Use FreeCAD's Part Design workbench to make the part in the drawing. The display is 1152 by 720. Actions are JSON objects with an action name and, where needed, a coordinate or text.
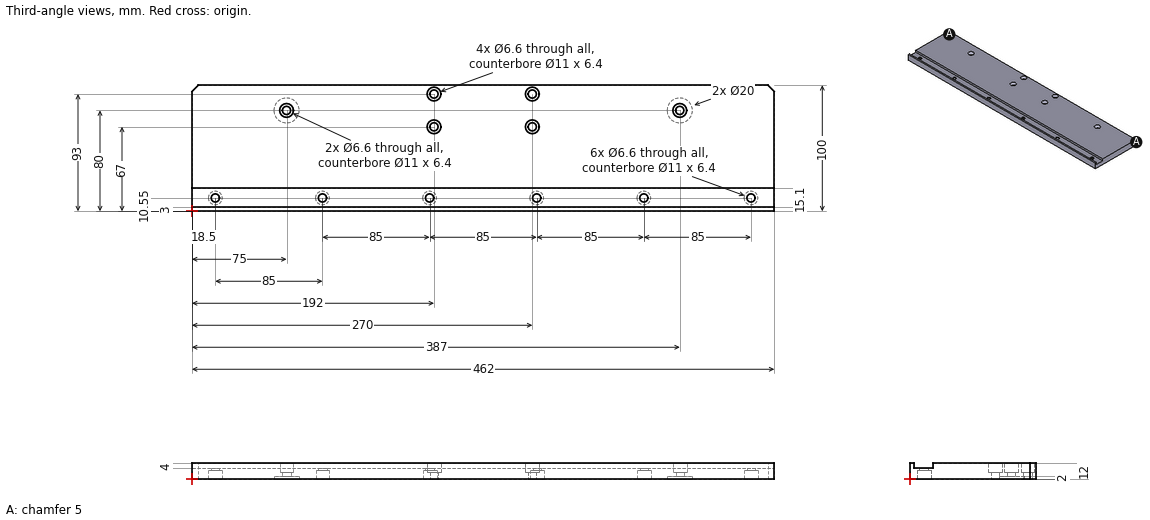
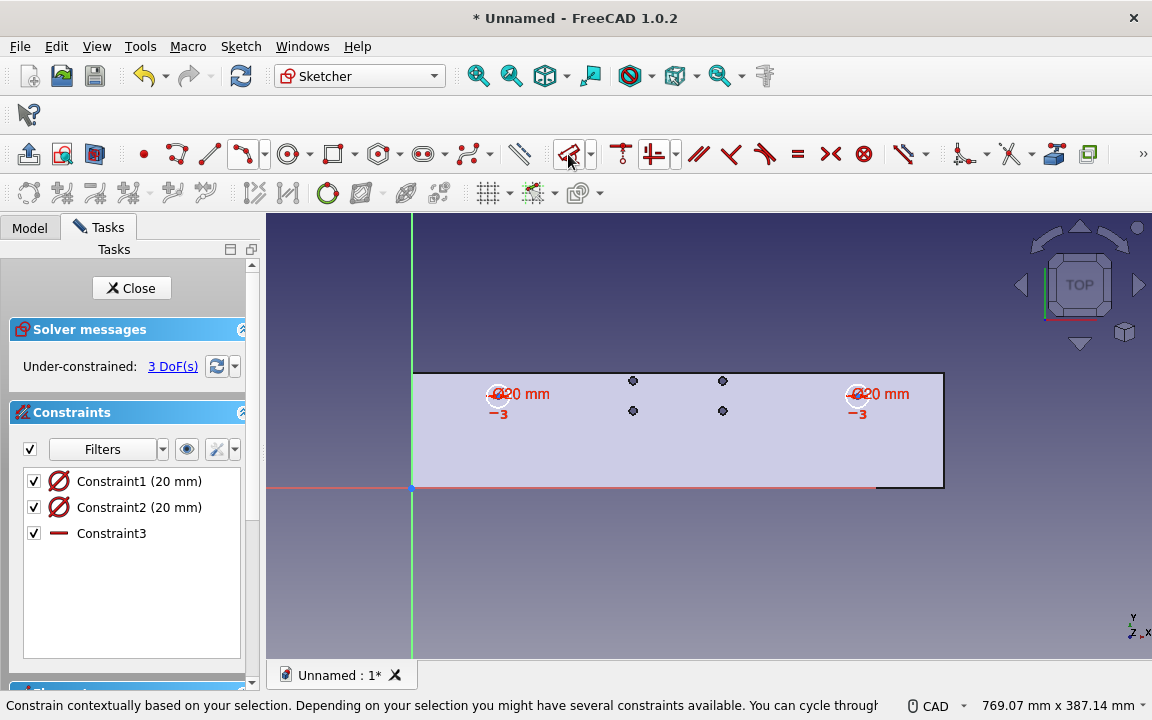
{"action": "left_click", "coordinate": [858, 396]}
{"action": "left_click", "coordinate": [378, 442]}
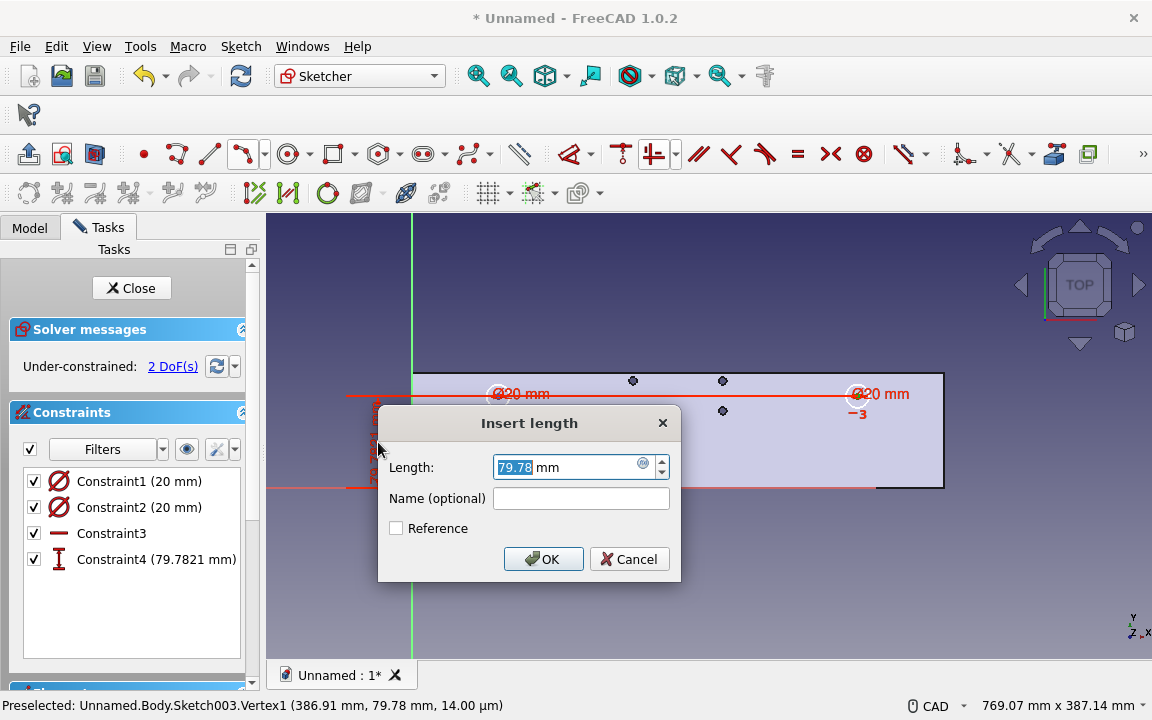
{"action": "type", "text": "80"}
{"action": "key", "text": "Return"}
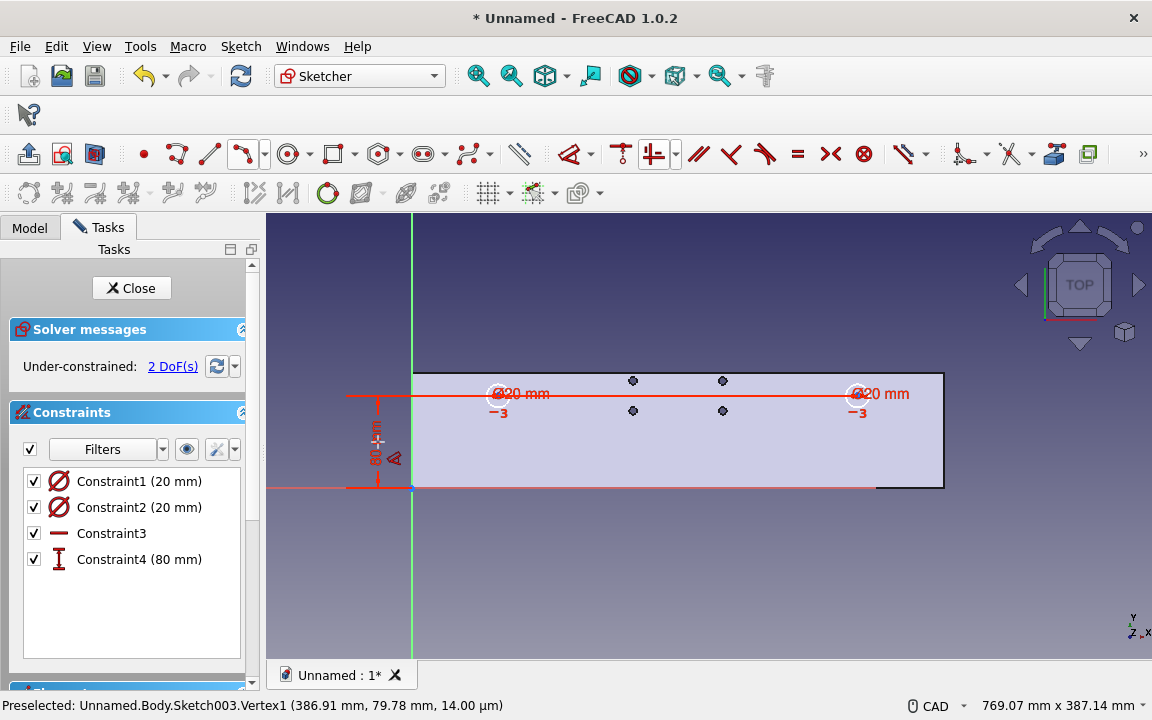
{"action": "left_click", "coordinate": [498, 396]}
{"action": "left_click", "coordinate": [455, 522]}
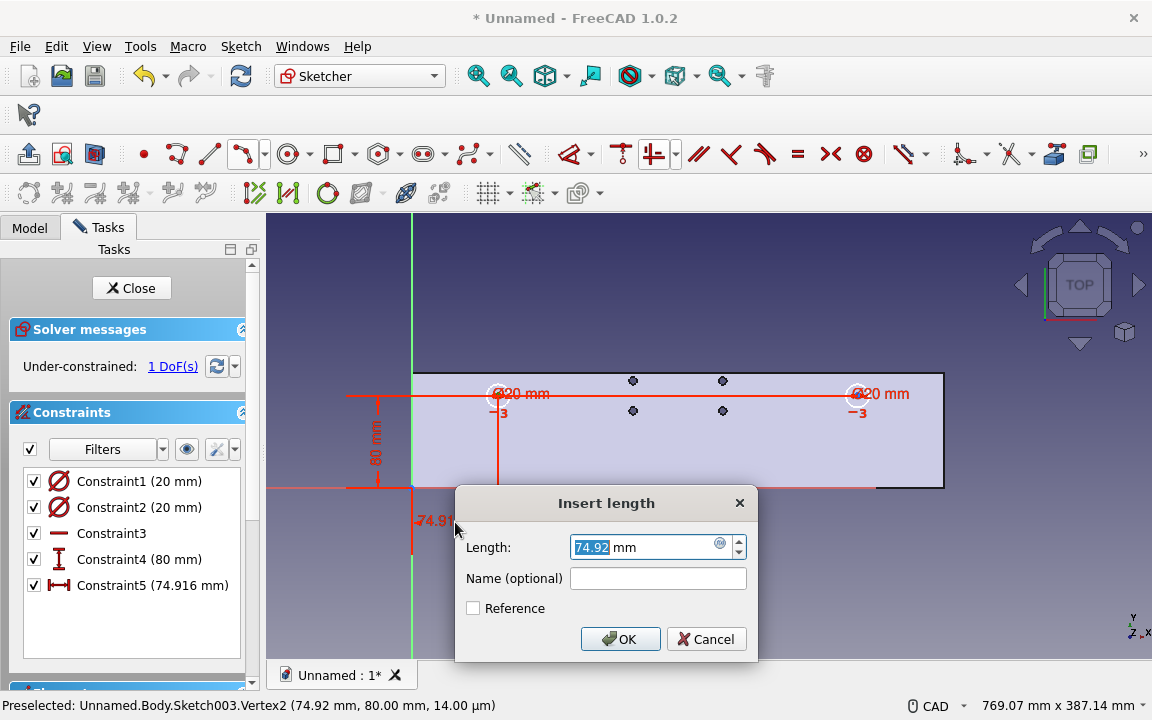
{"action": "type", "text": "75"}
{"action": "key", "text": "Return"}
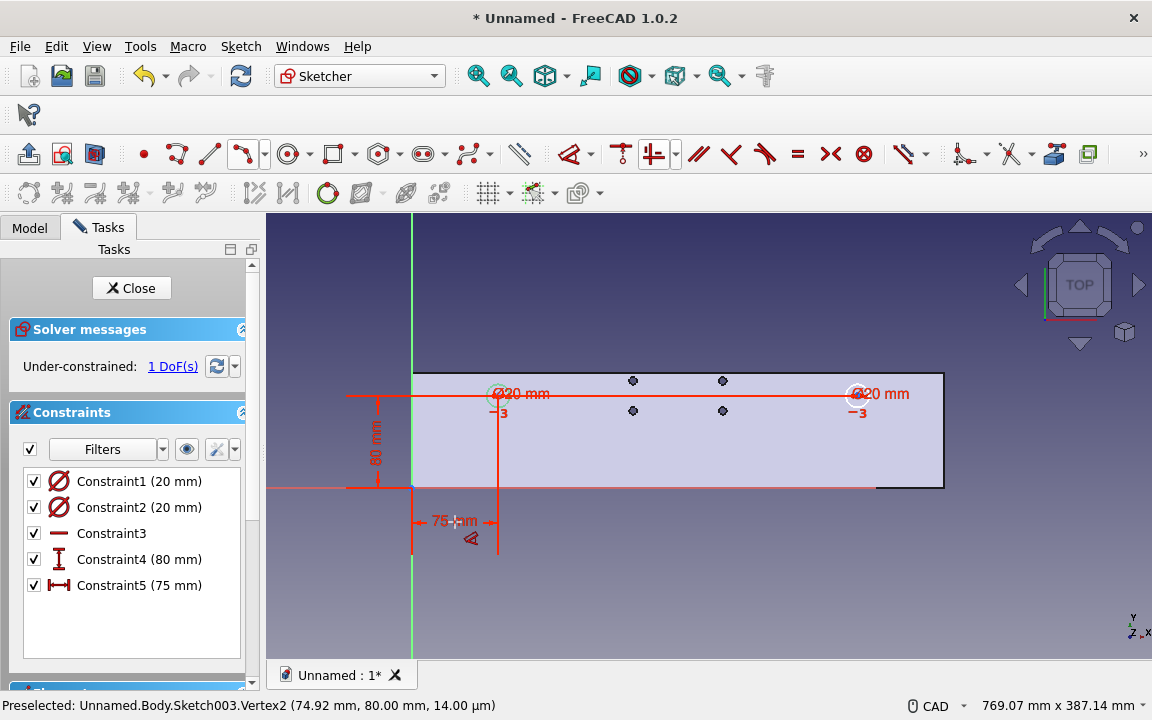
{"action": "left_click", "coordinate": [858, 396]}
{"action": "left_click", "coordinate": [635, 522]}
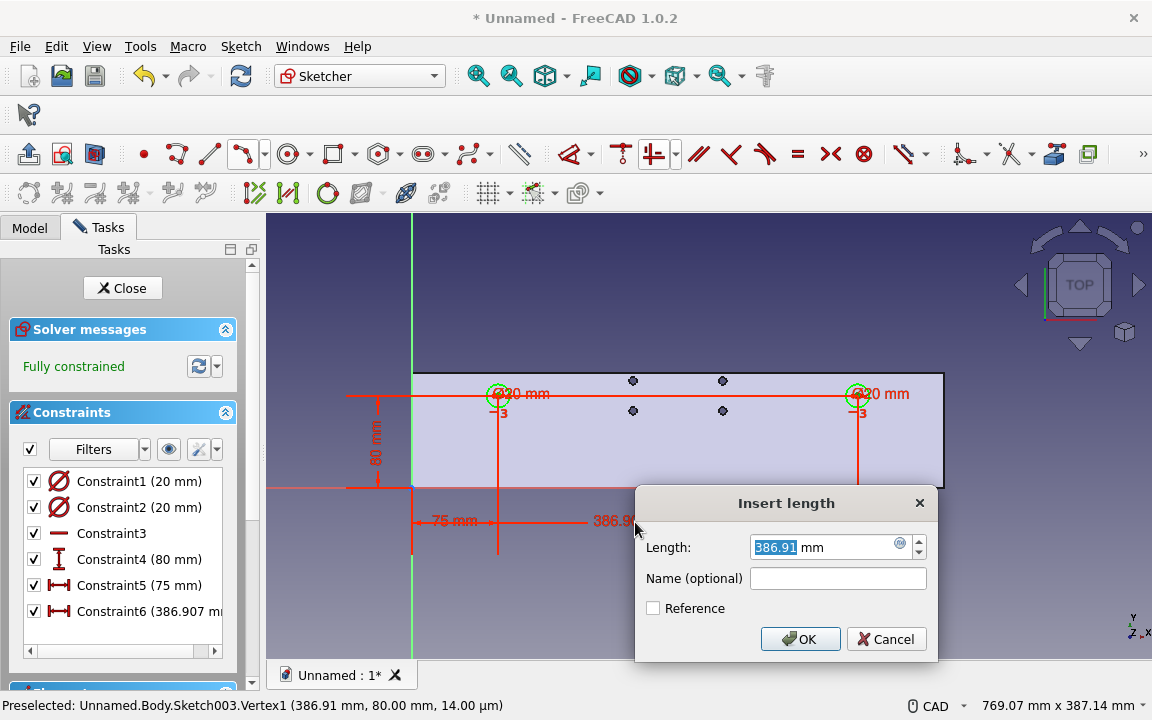
{"action": "type", "text": "387"}
{"action": "key", "text": "Return"}
{"action": "key", "text": "Escape"}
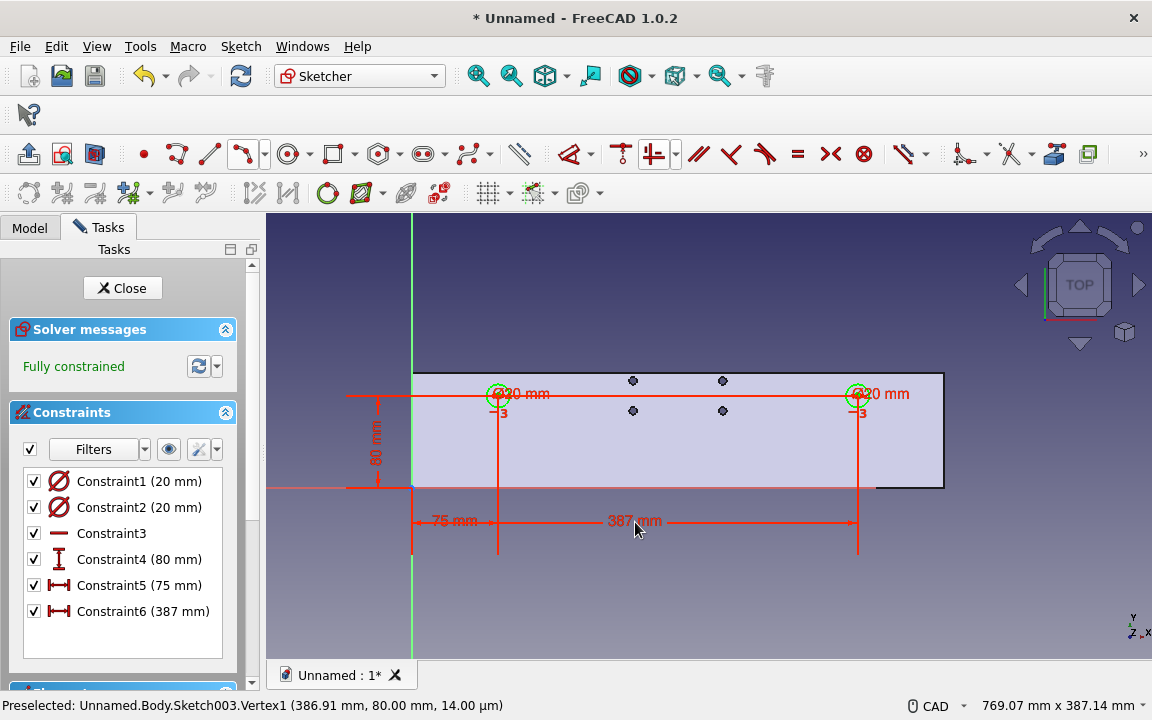
{"action": "left_click", "coordinate": [123, 288]}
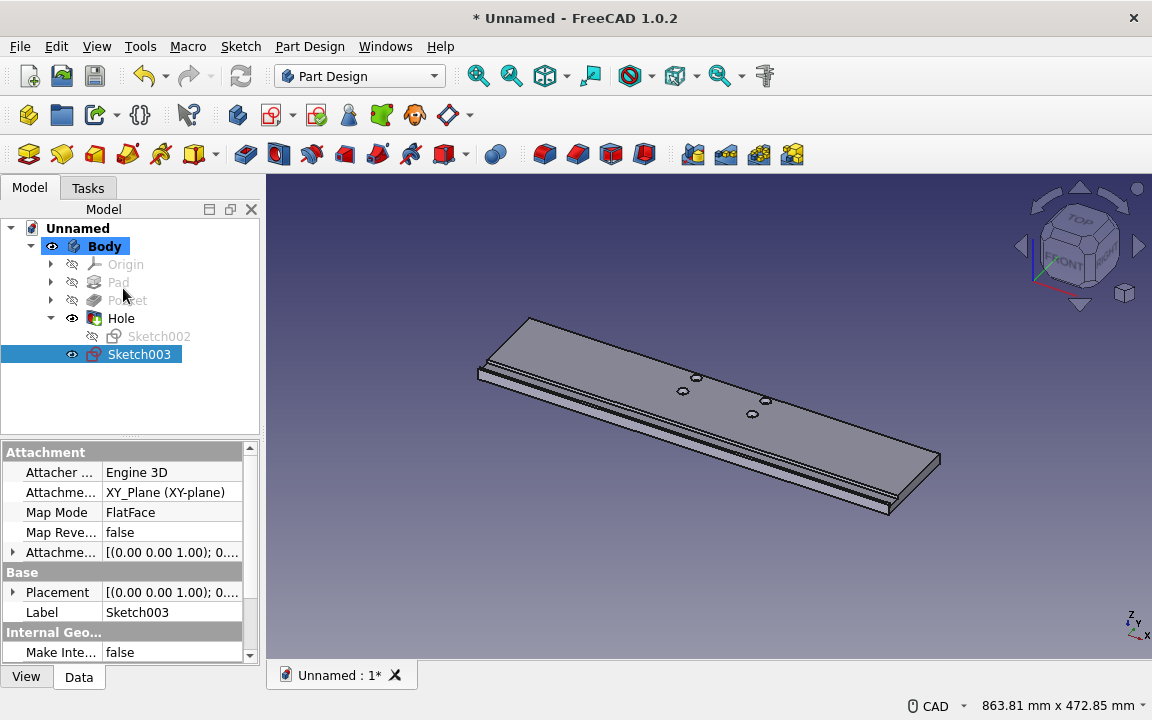
{"action": "left_click", "coordinate": [246, 154]}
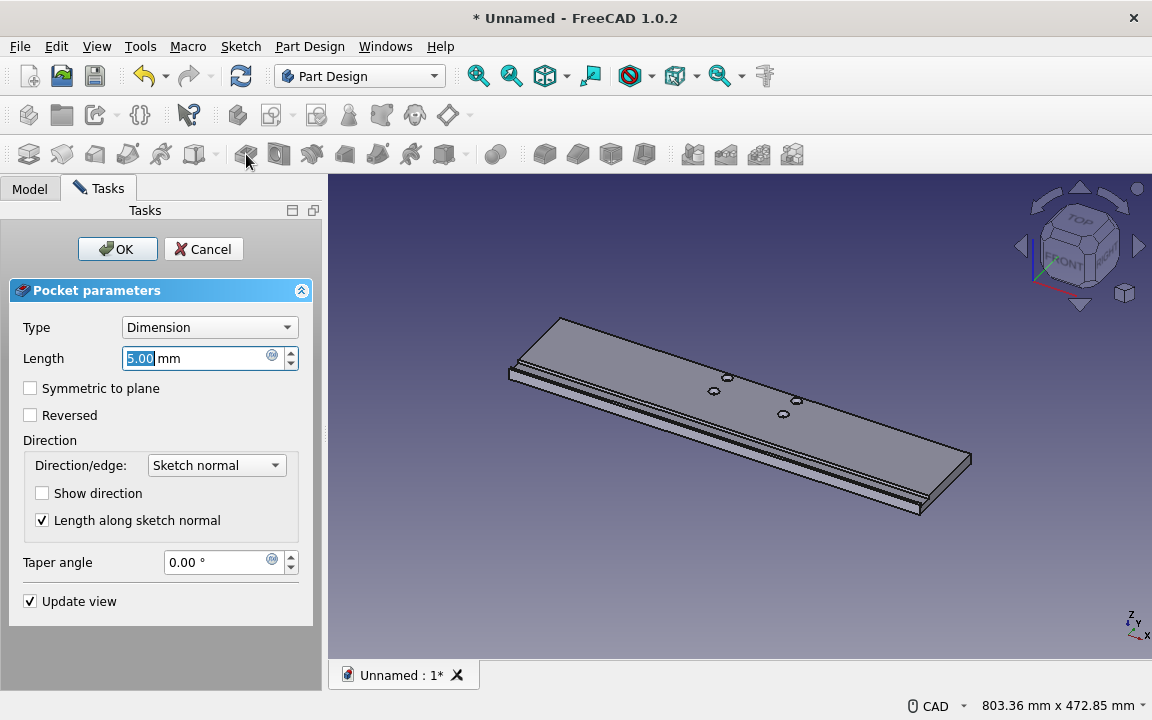
{"action": "type", "text": "2"}
{"action": "key", "text": "Tab"}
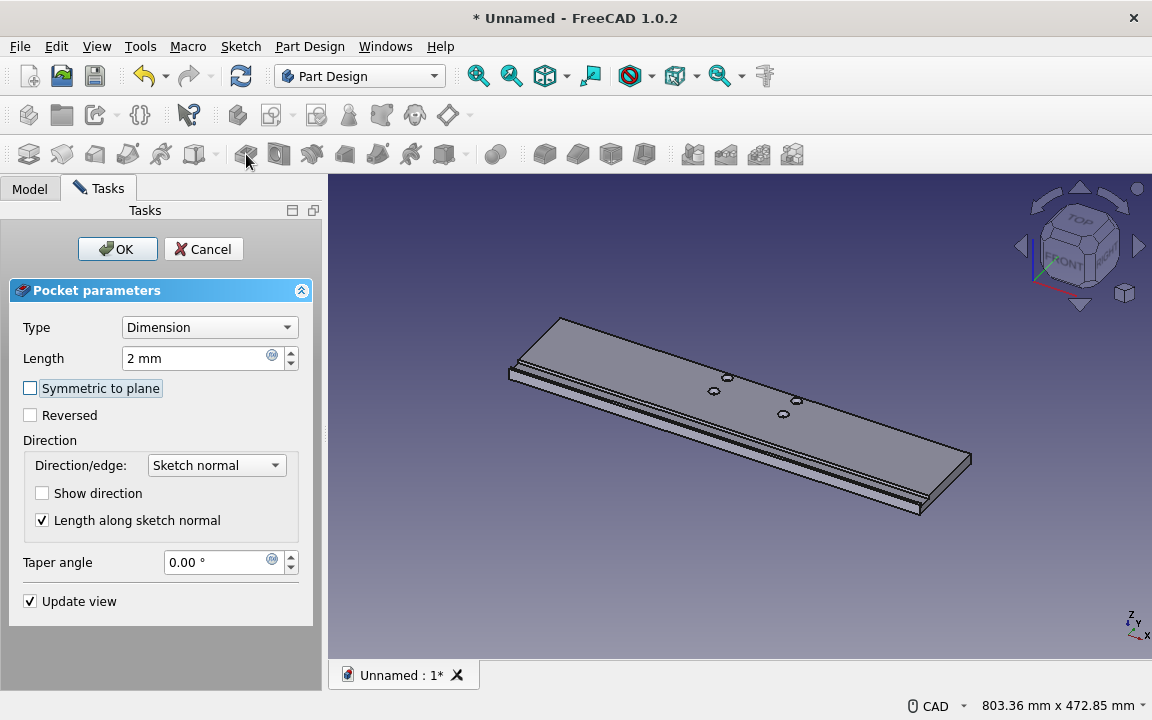
{"action": "left_click", "coordinate": [31, 415]}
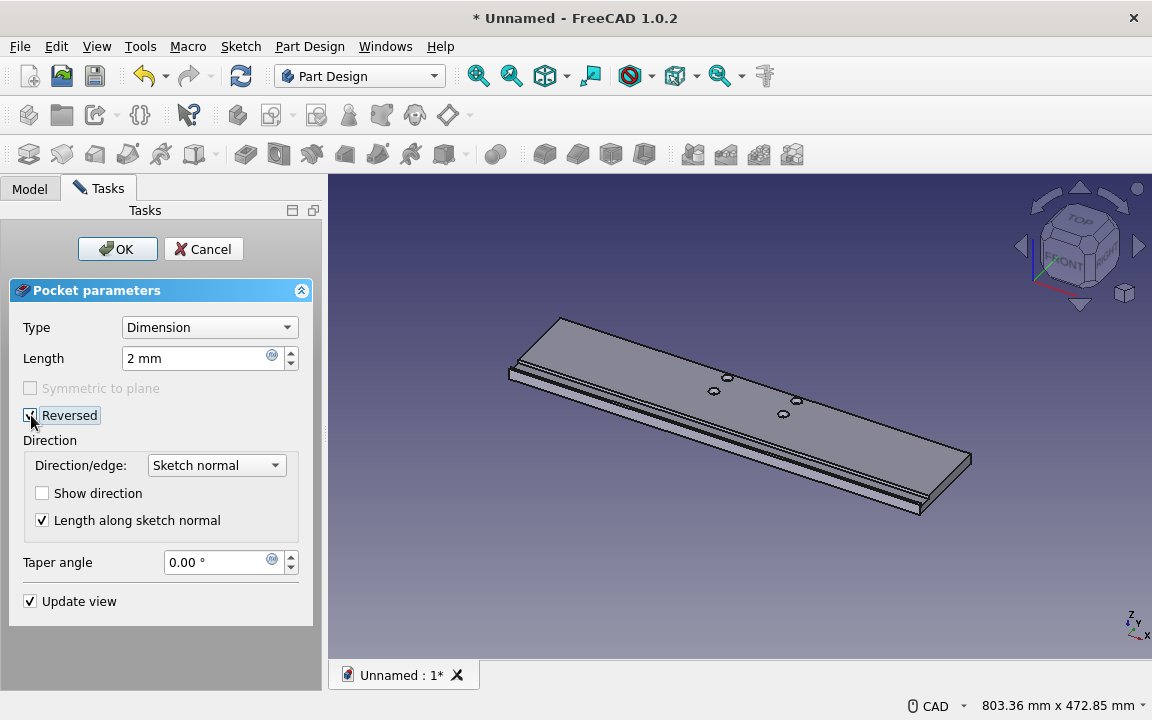
{"action": "left_click", "coordinate": [118, 249]}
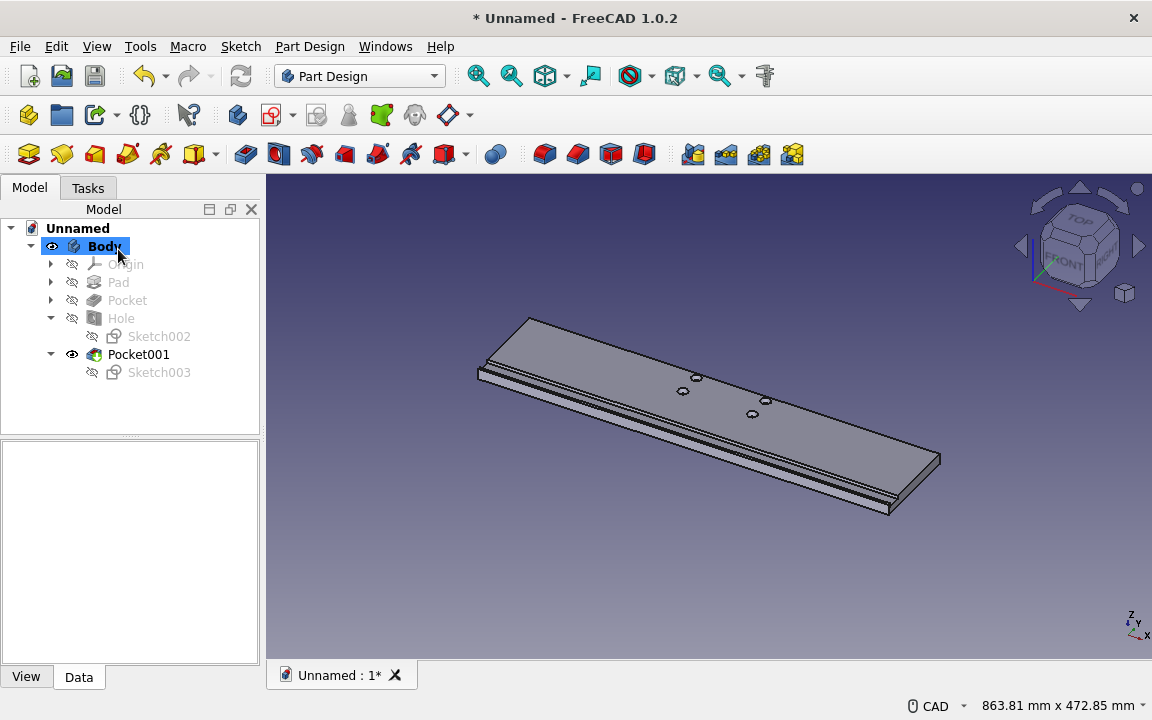
{"action": "left_click", "coordinate": [831, 445]}